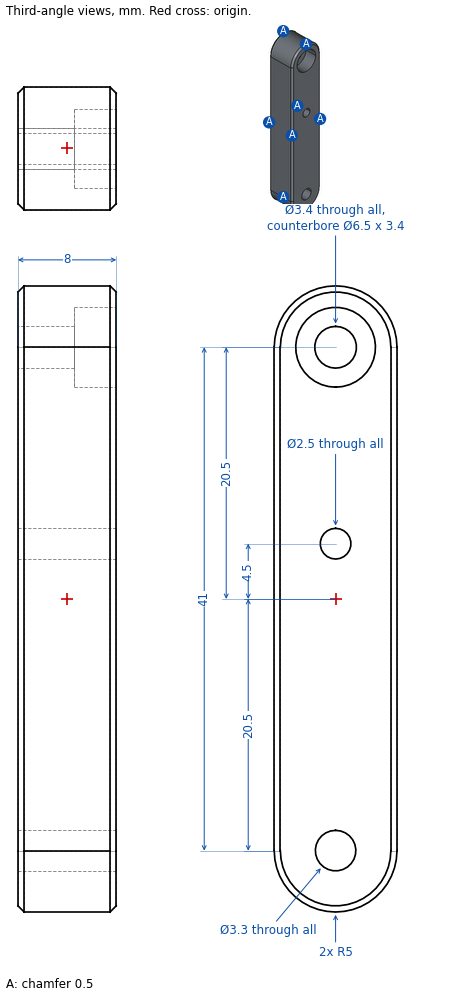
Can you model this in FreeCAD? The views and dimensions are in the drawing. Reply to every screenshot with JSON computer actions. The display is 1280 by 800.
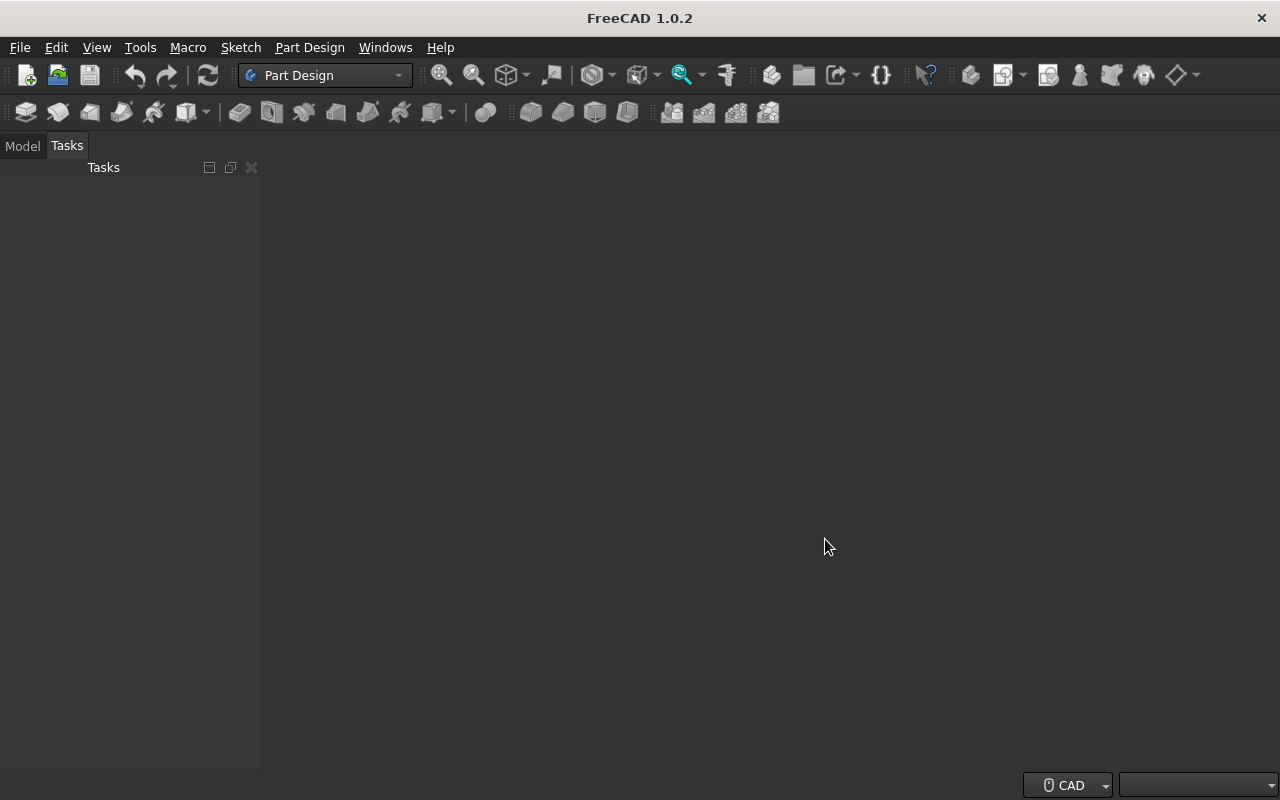
{"action": "key", "text": "ctrl+n"}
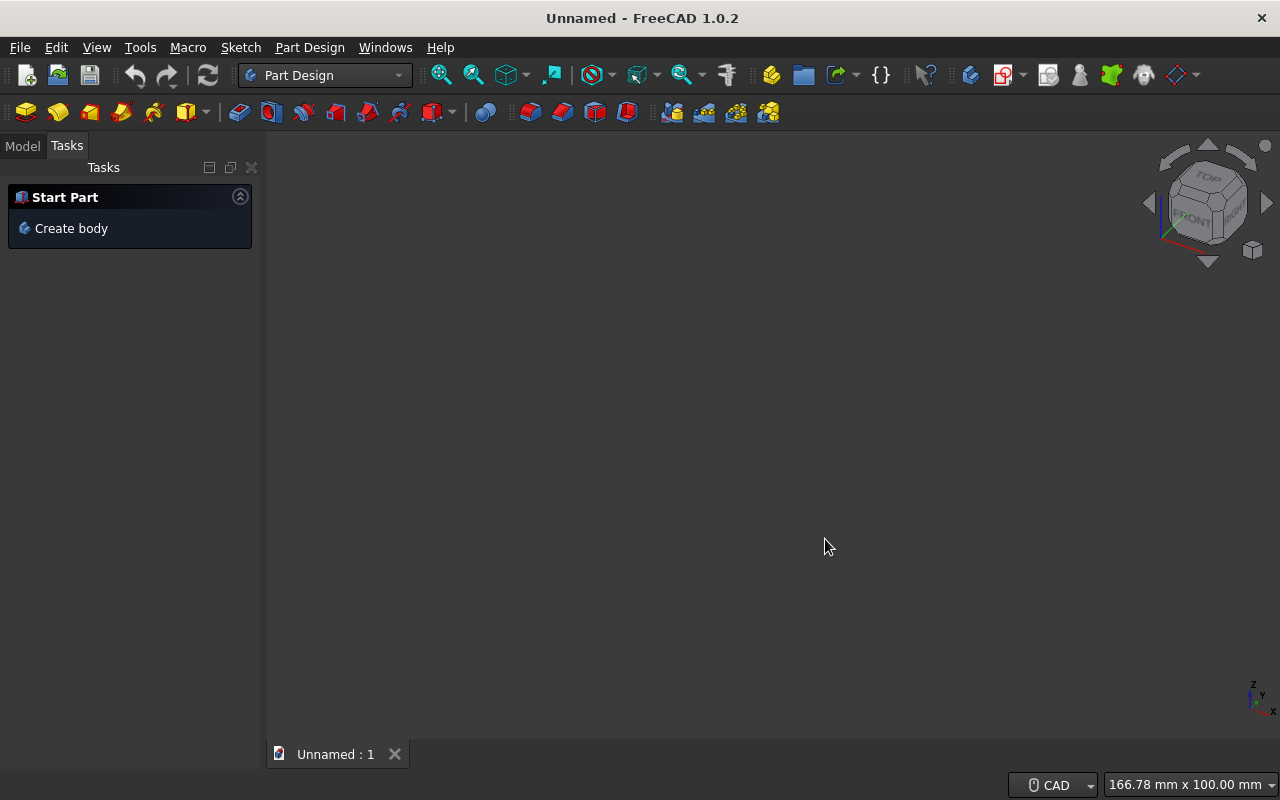
{"action": "left_click", "coordinate": [1004, 76]}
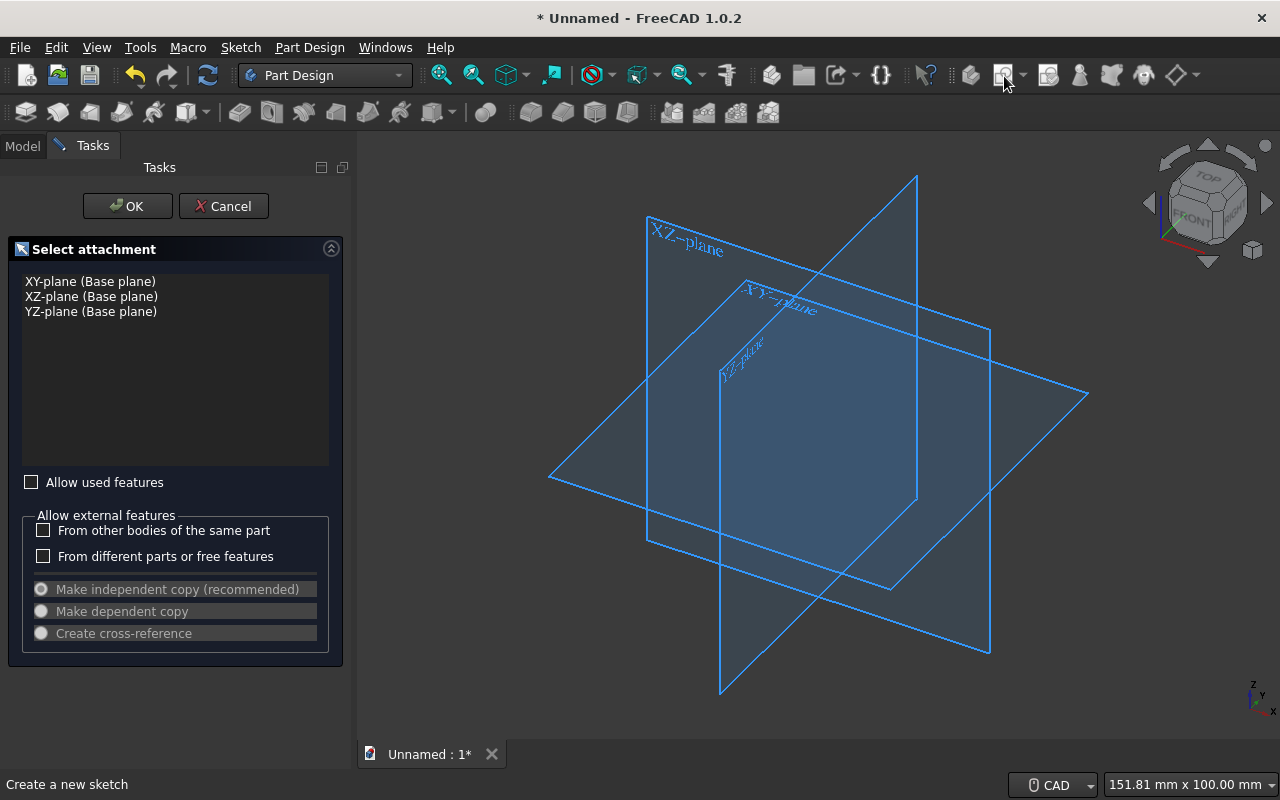
{"action": "left_click", "coordinate": [82, 312]}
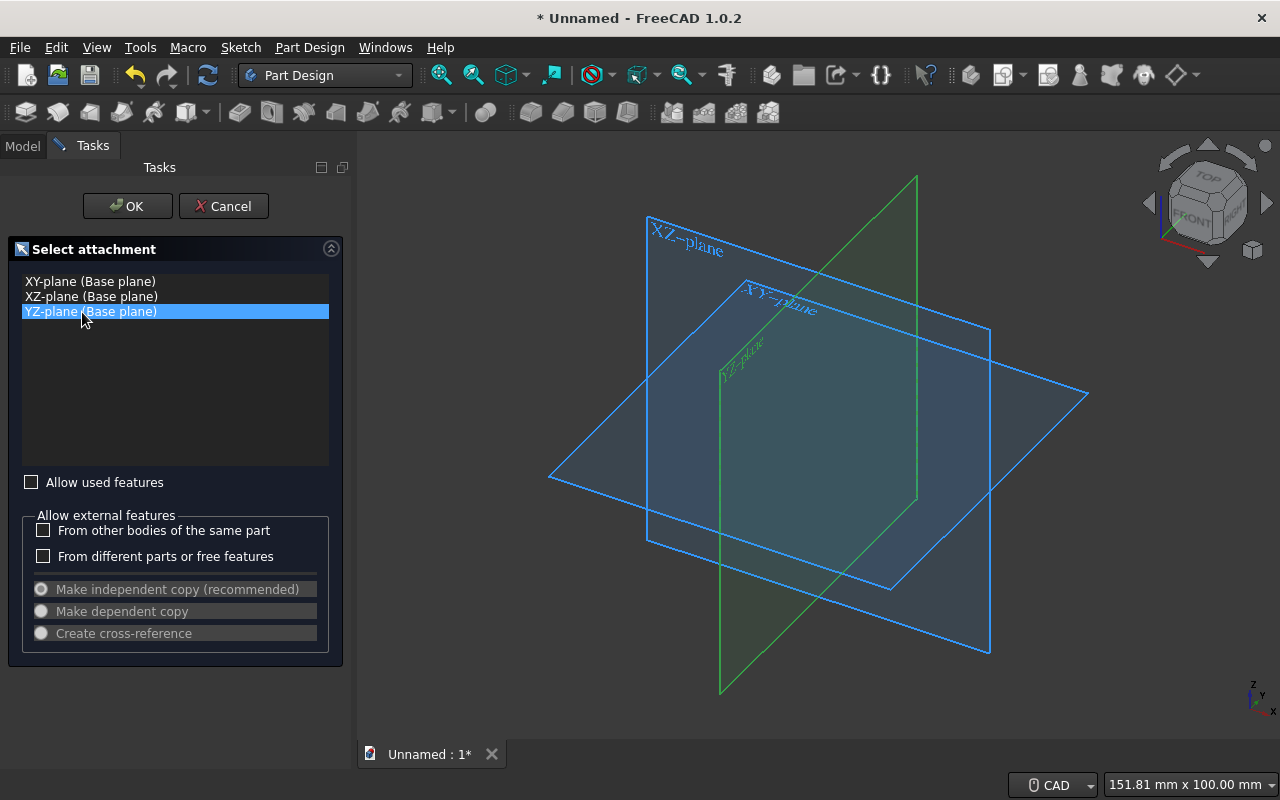
{"action": "left_click", "coordinate": [128, 206]}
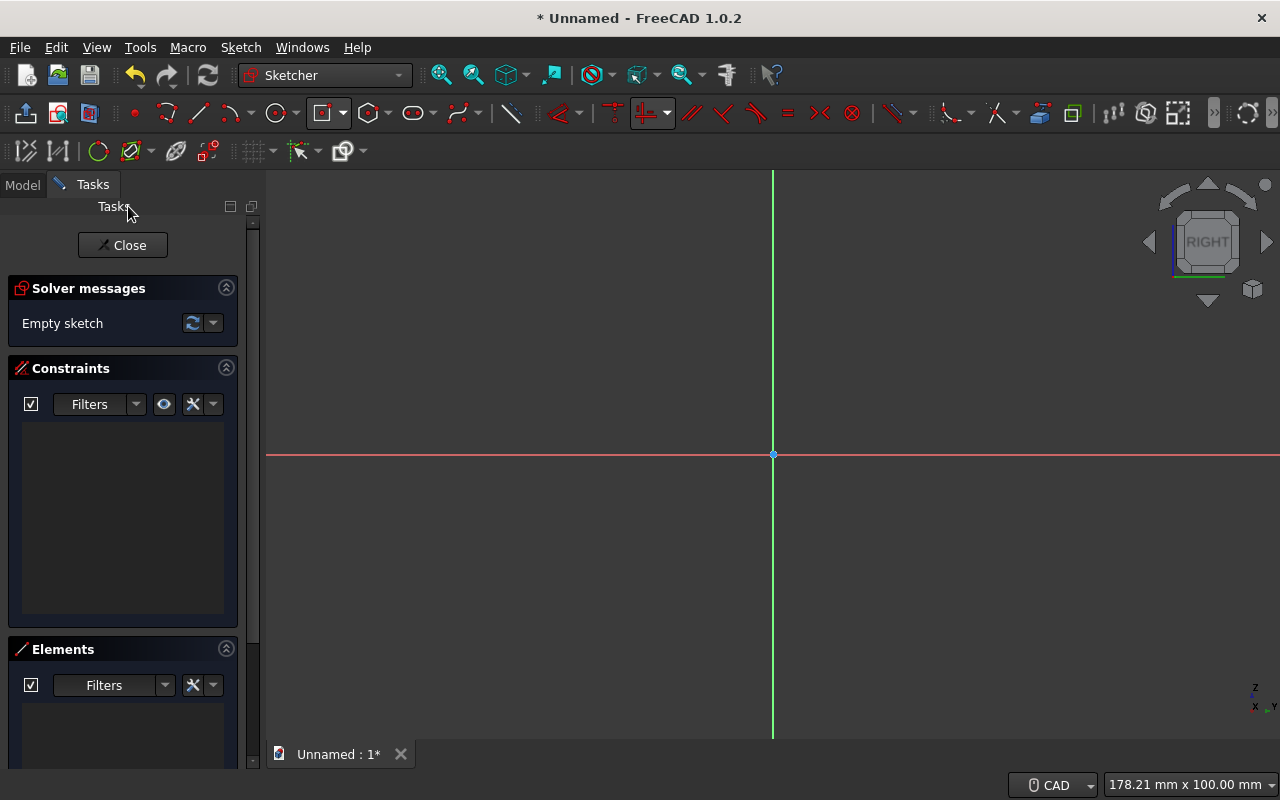
{"action": "left_click", "coordinate": [414, 114]}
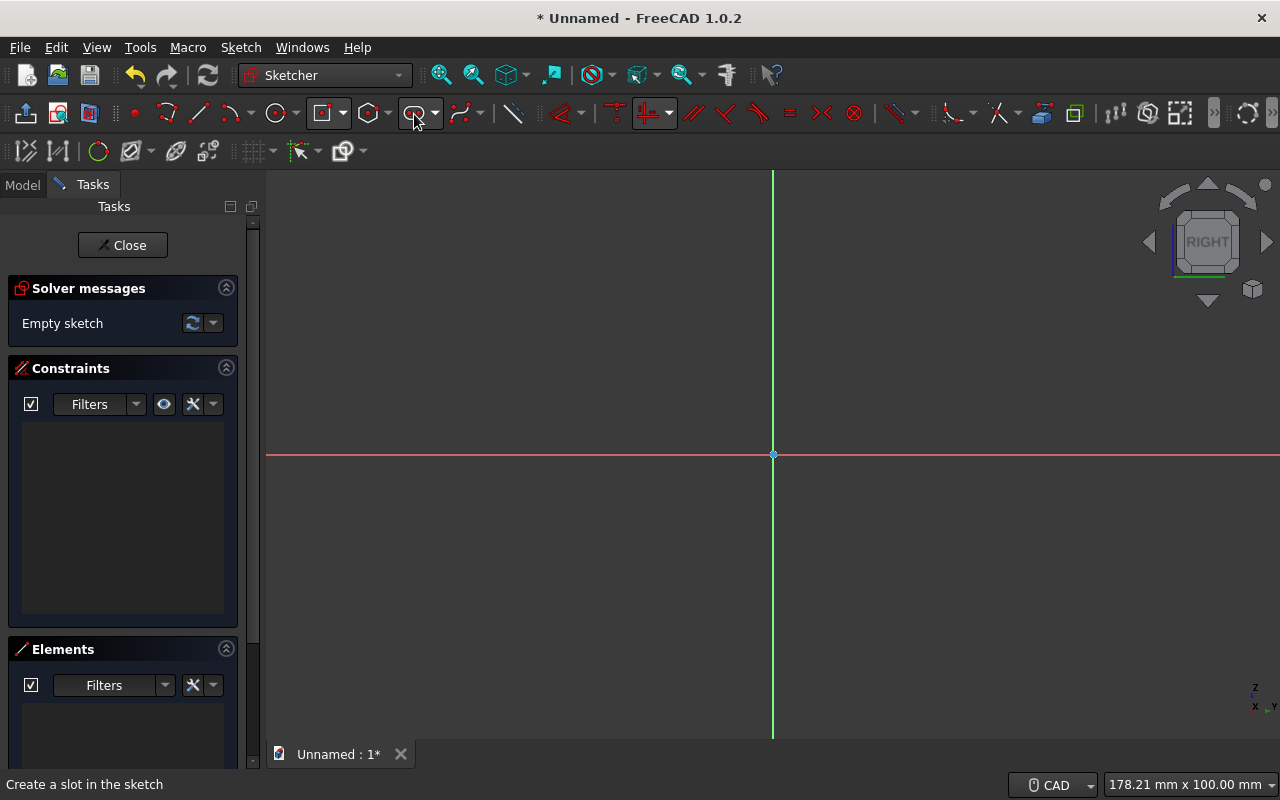
{"action": "left_click", "coordinate": [773, 571]}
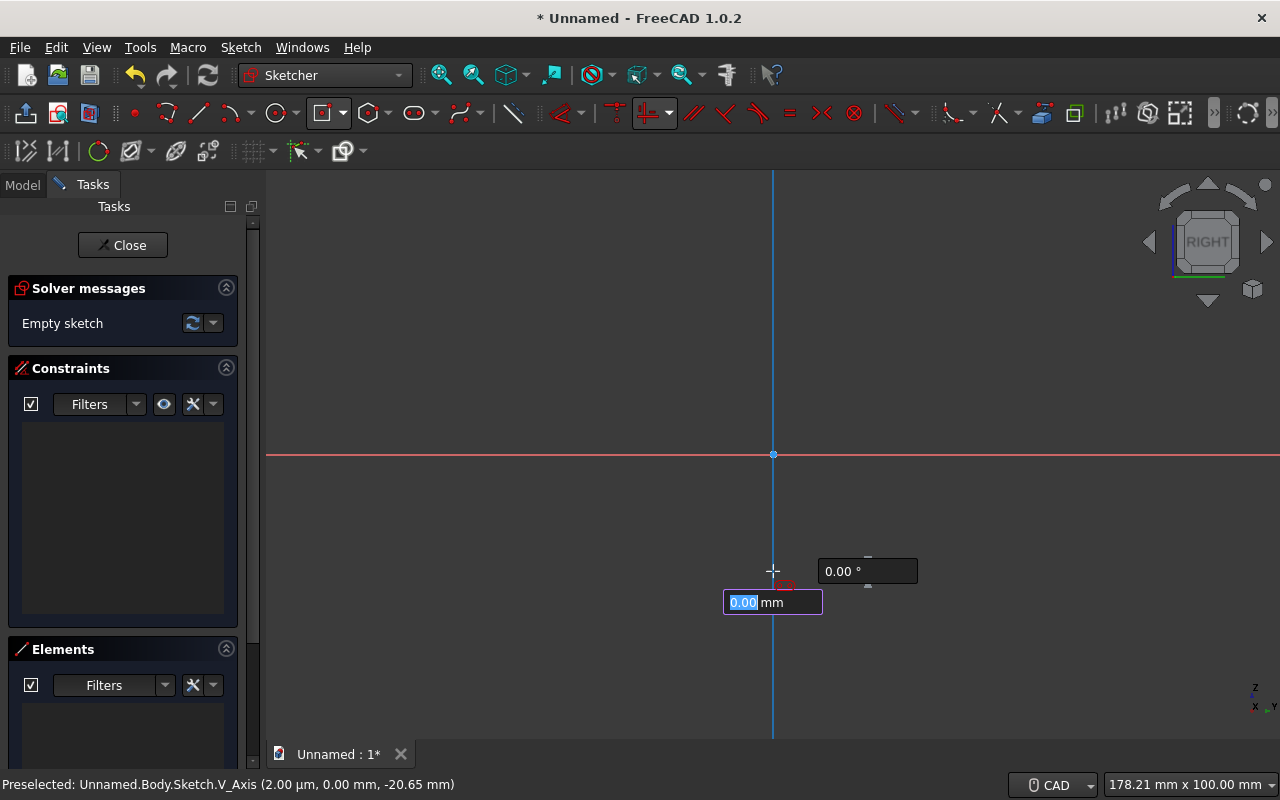
{"action": "left_click", "coordinate": [782, 338]}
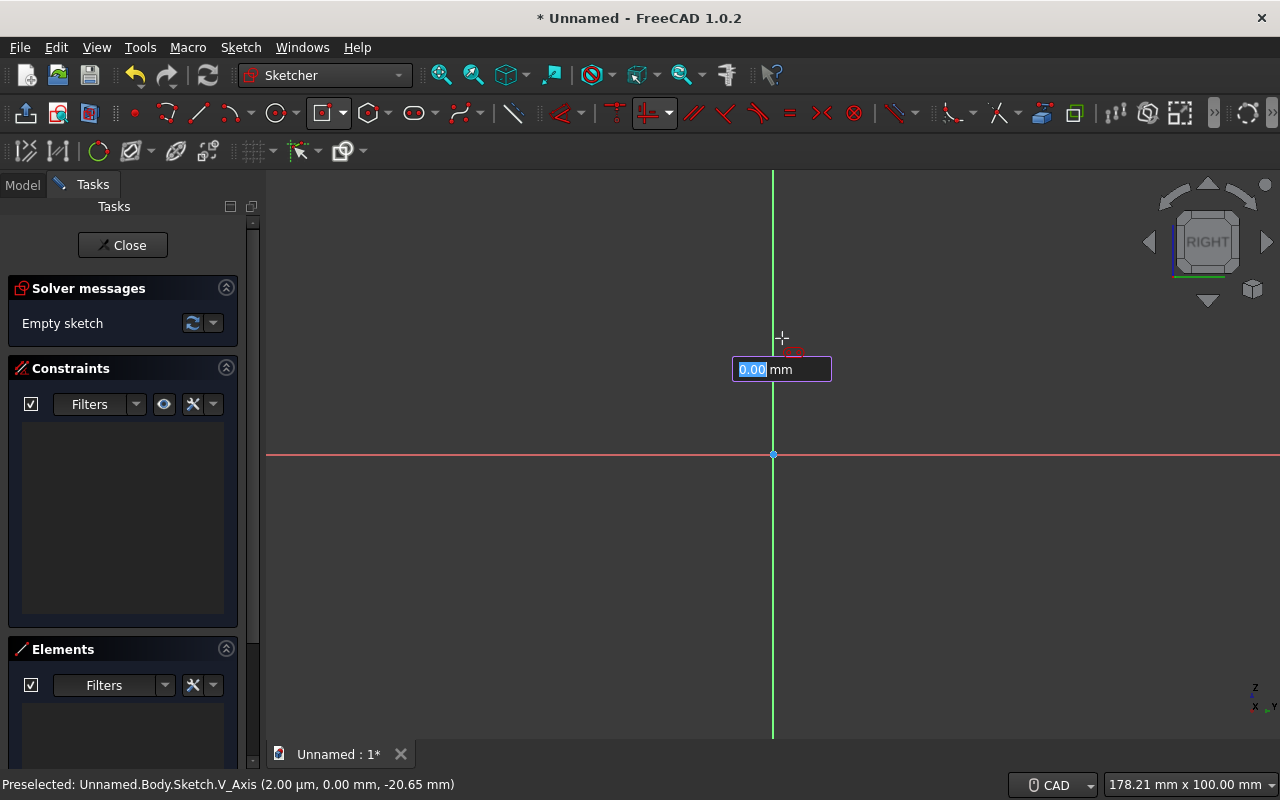
{"action": "left_click", "coordinate": [745, 420]}
{"action": "key", "text": "Escape"}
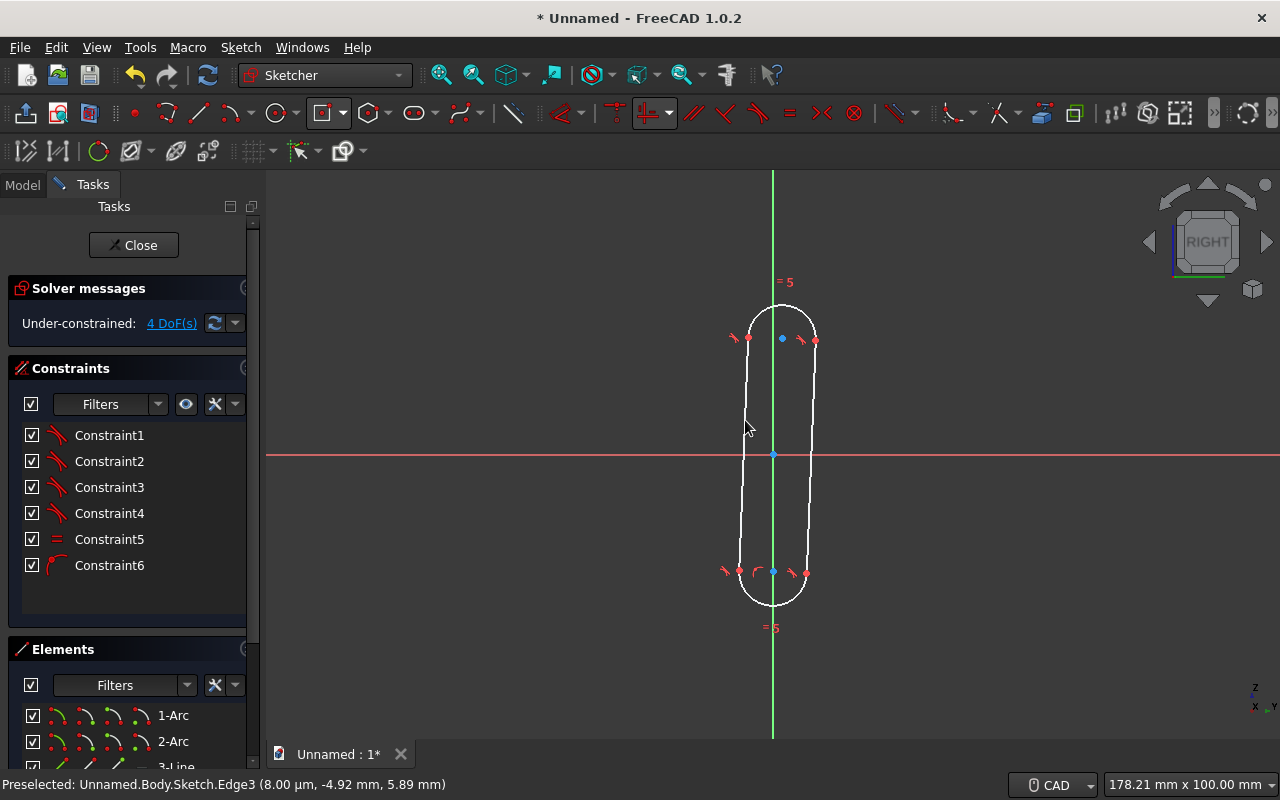
{"action": "left_click", "coordinate": [742, 501]}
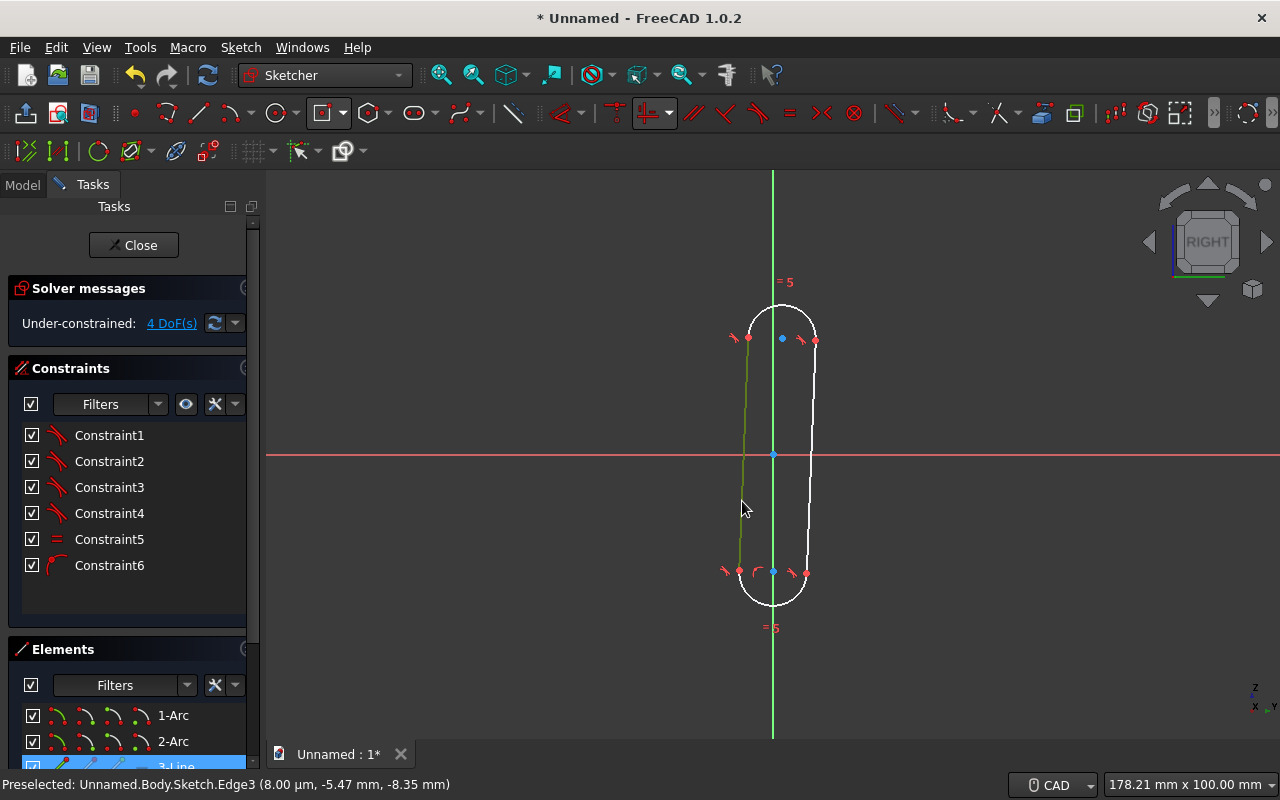
{"action": "left_click", "coordinate": [672, 114]}